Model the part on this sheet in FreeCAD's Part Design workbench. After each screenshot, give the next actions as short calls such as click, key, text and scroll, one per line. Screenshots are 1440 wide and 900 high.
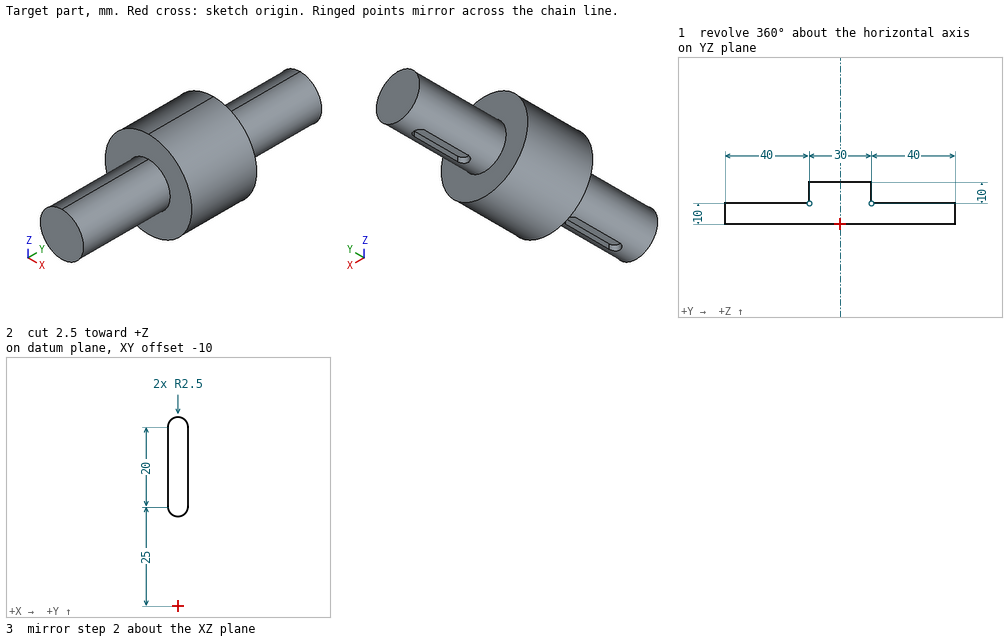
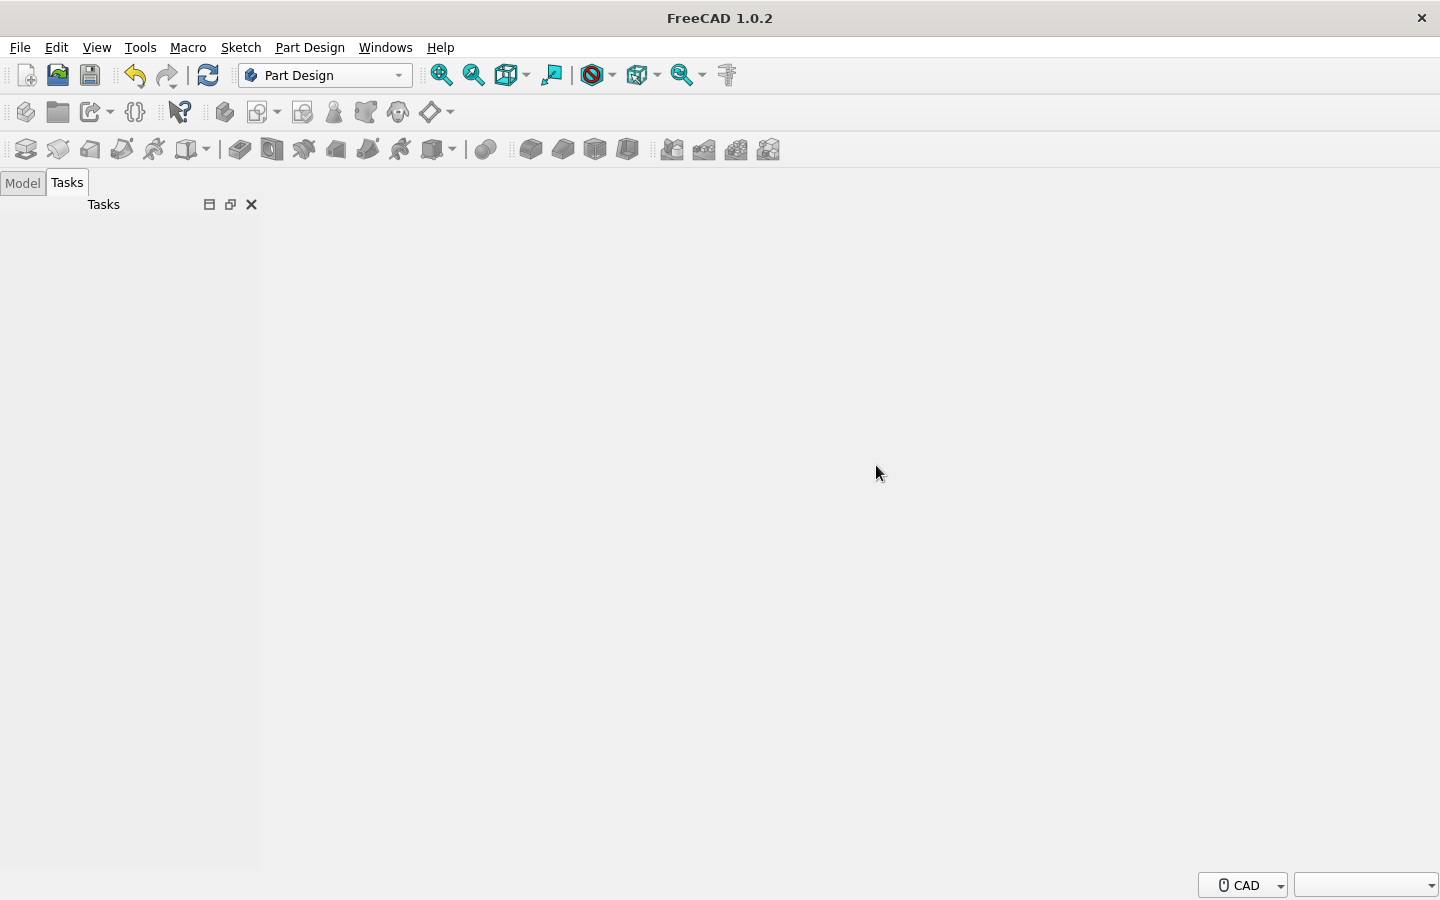
click(26, 76)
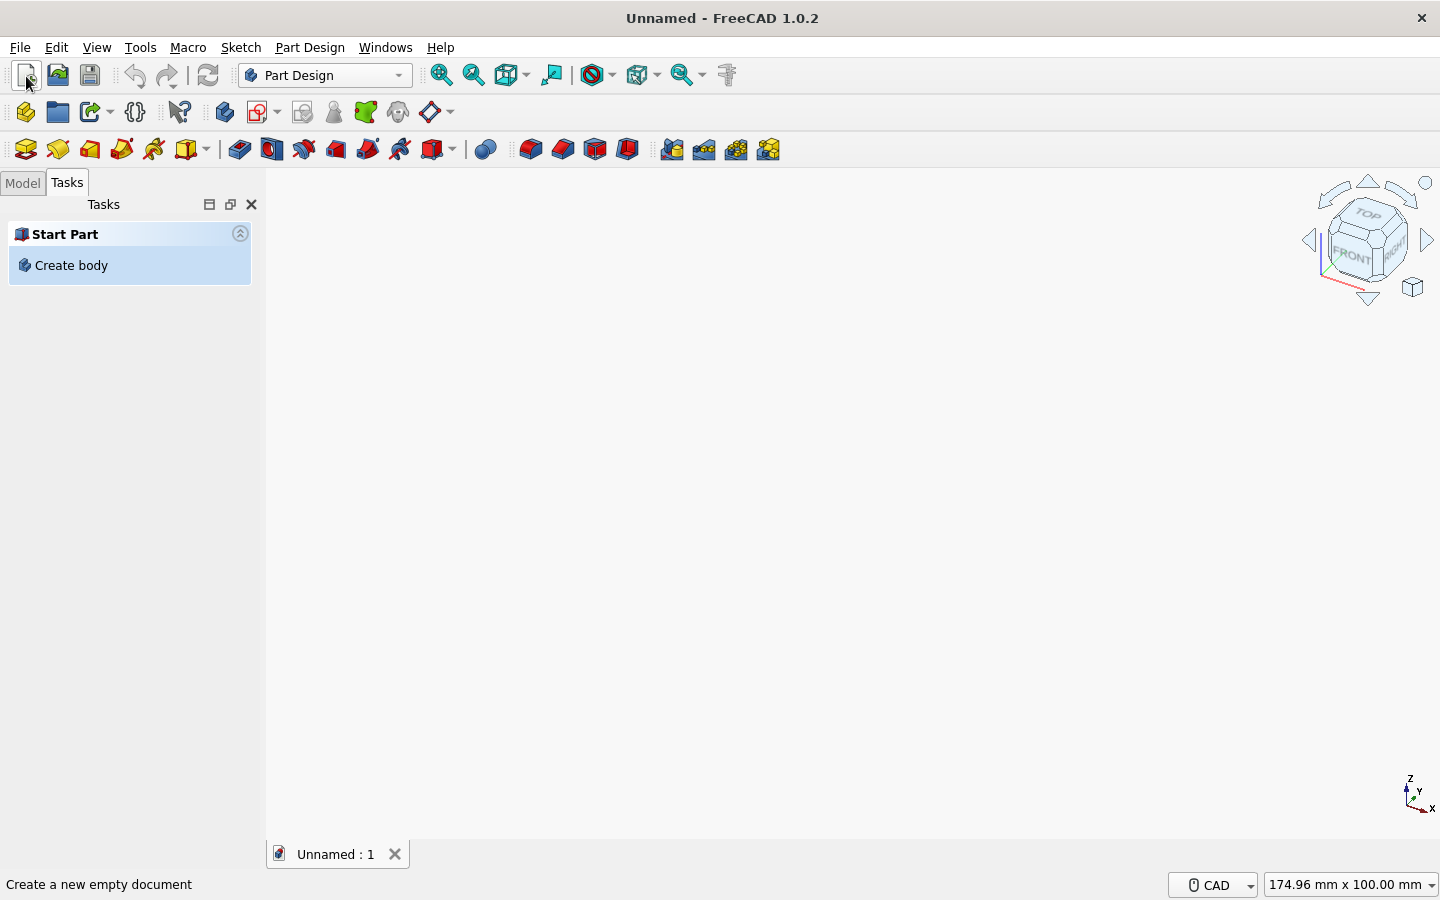
click(258, 112)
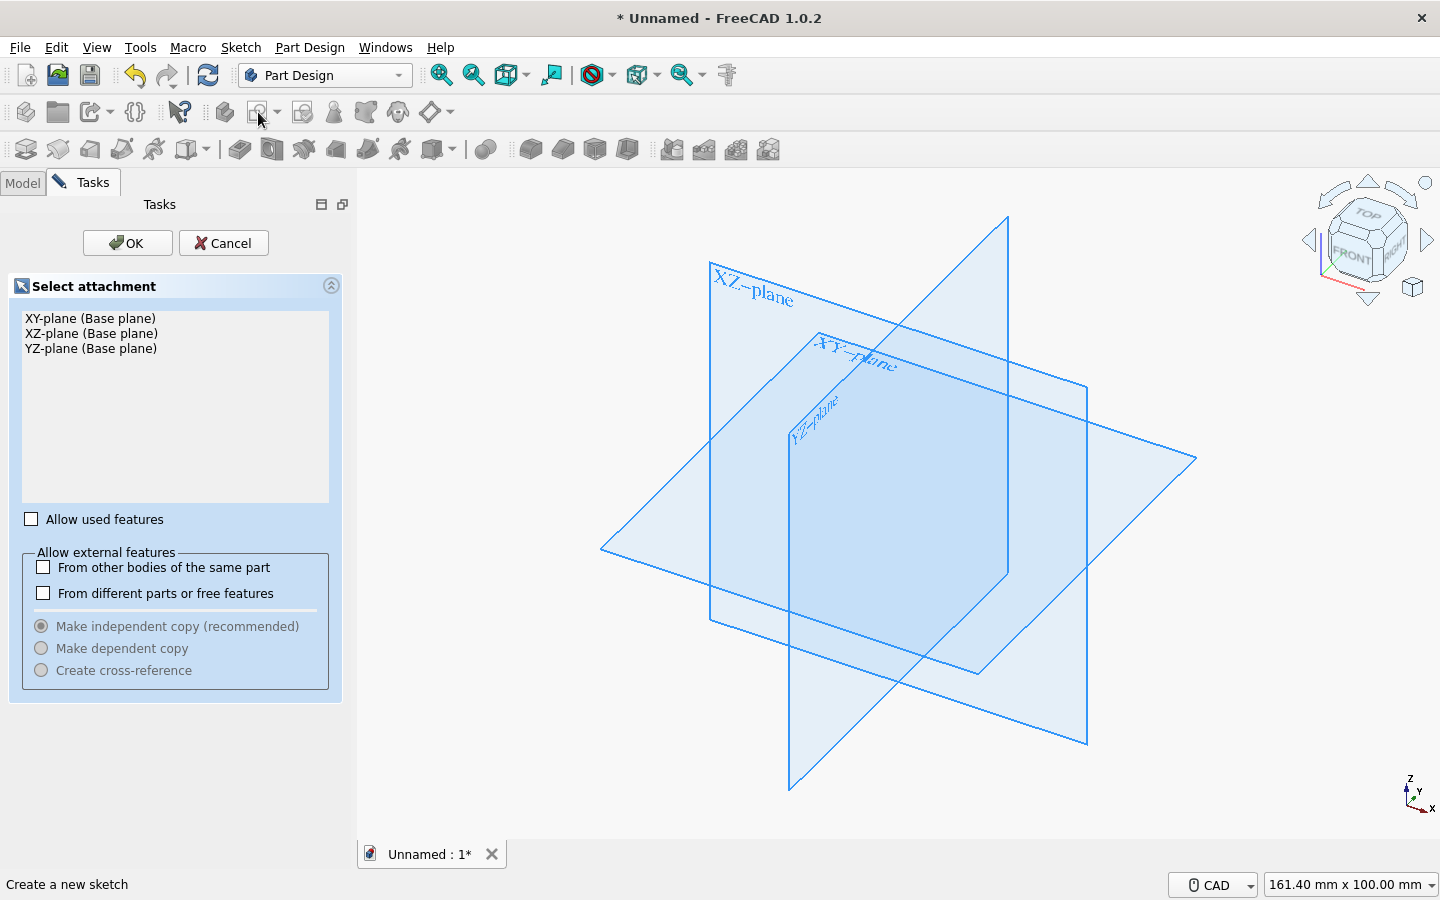
click(82, 348)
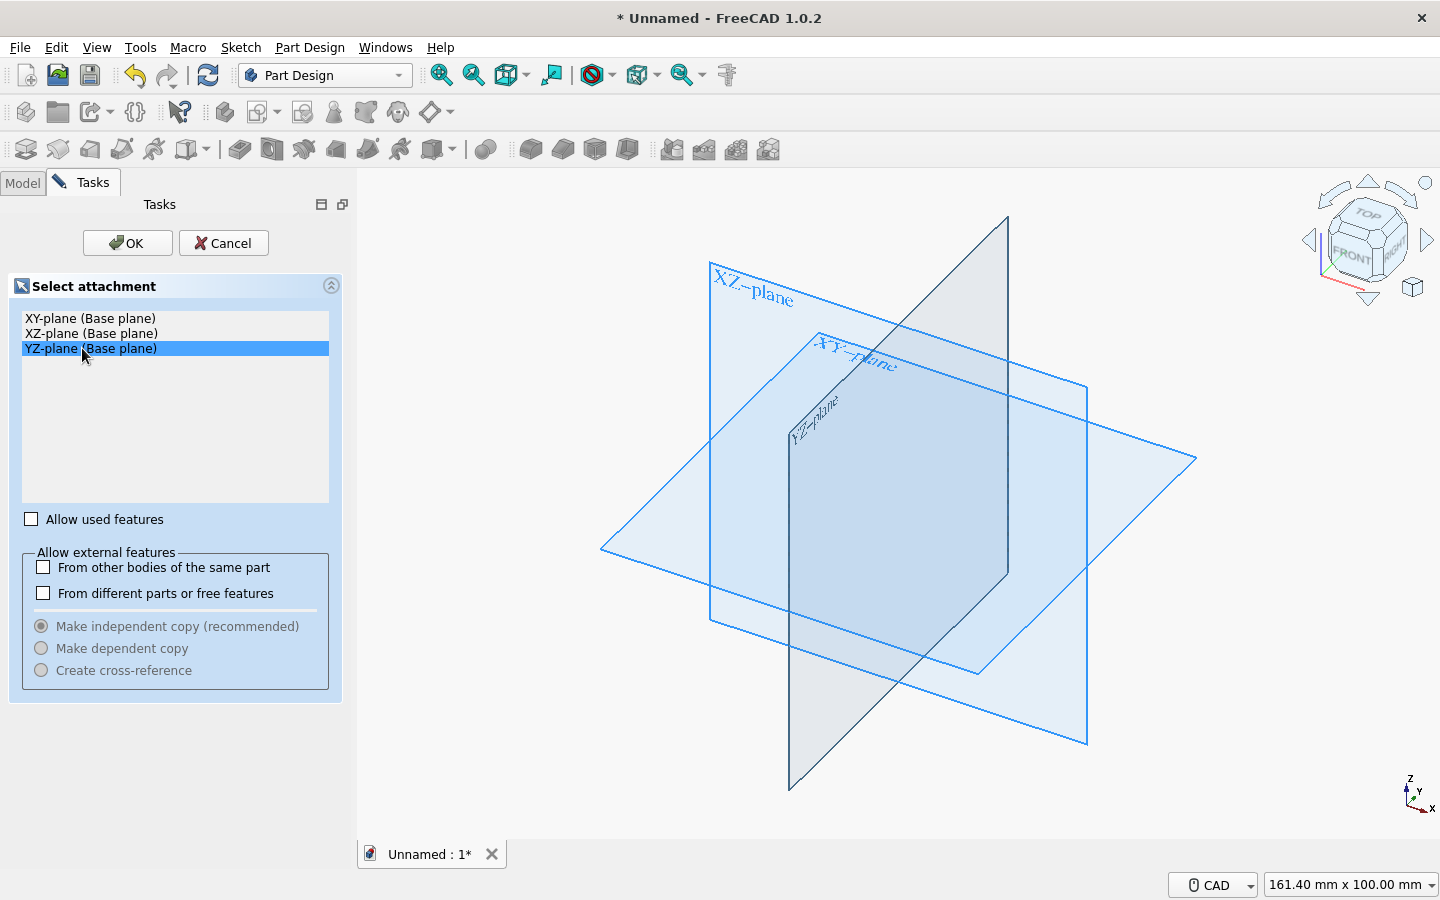
click(128, 243)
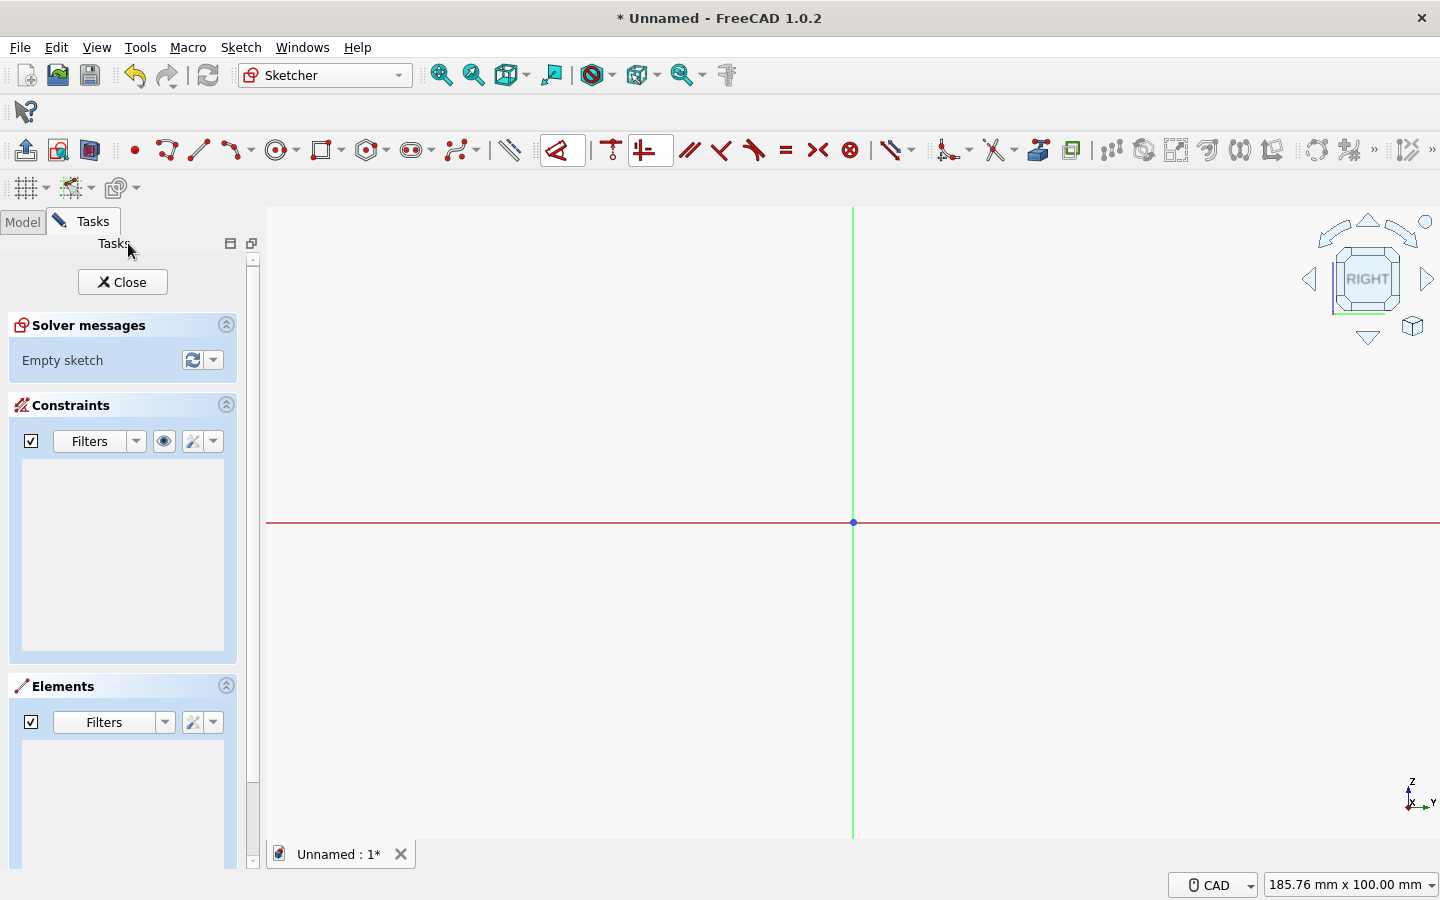
click(168, 150)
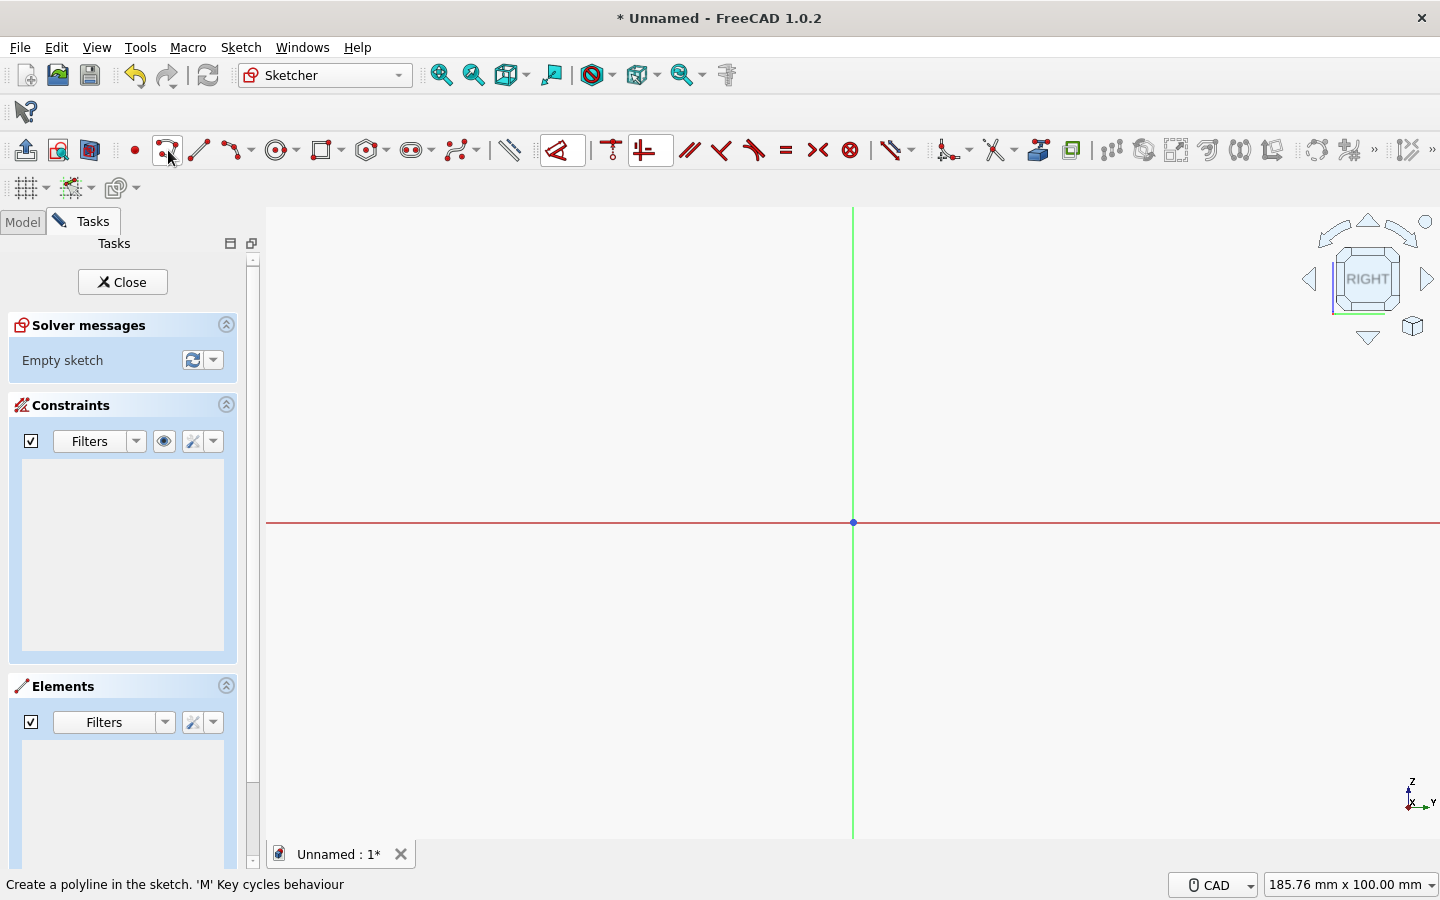
click(948, 460)
click(948, 397)
click(758, 397)
click(758, 460)
click(505, 460)
click(505, 523)
click(1201, 514)
click(1201, 460)
click(948, 461)
key(Escape)
key(Escape)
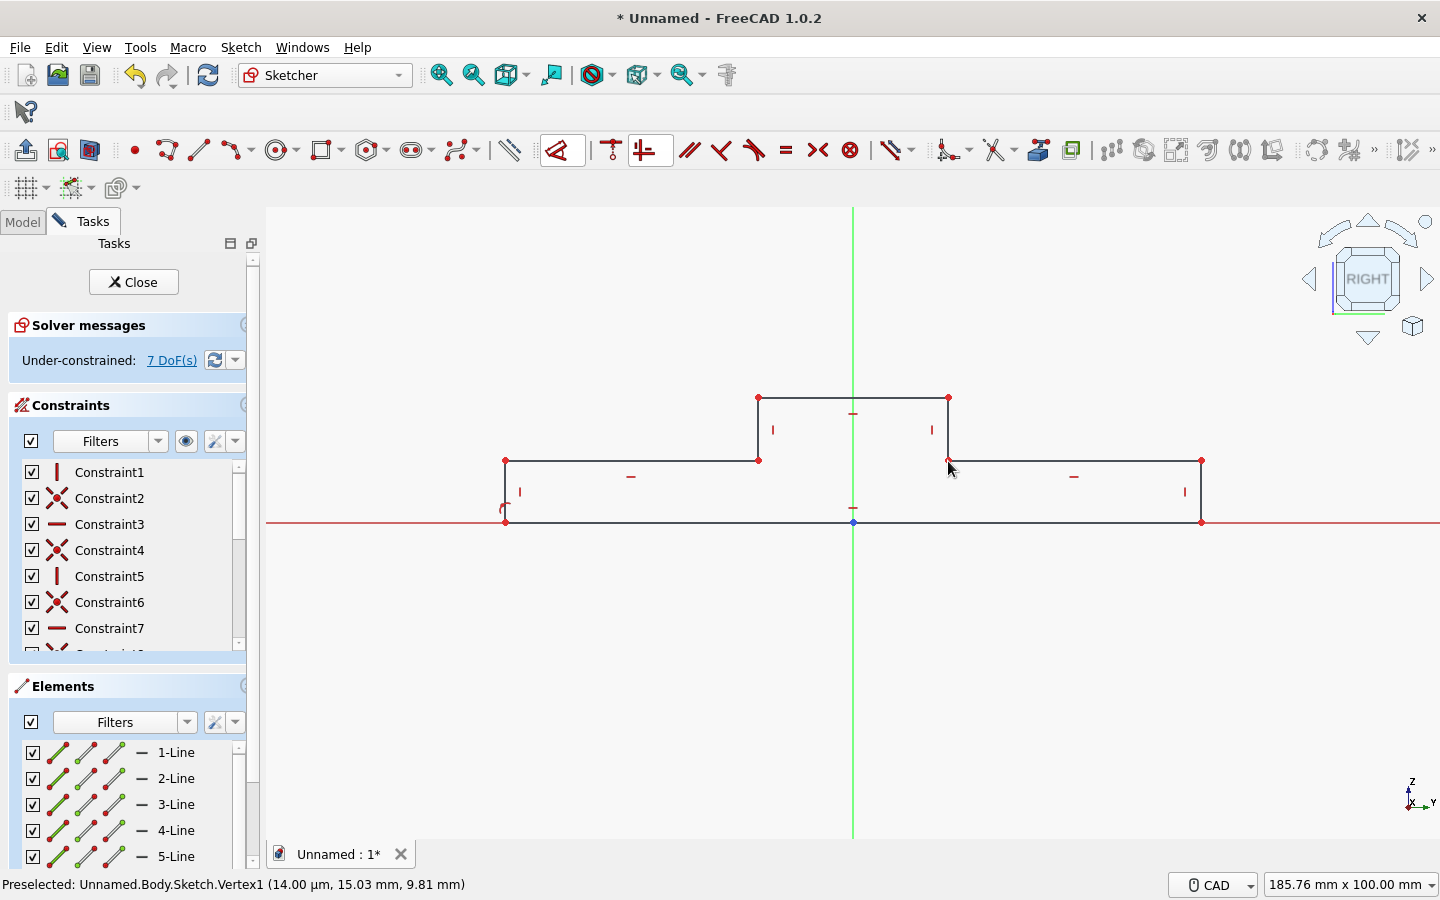
click(948, 461)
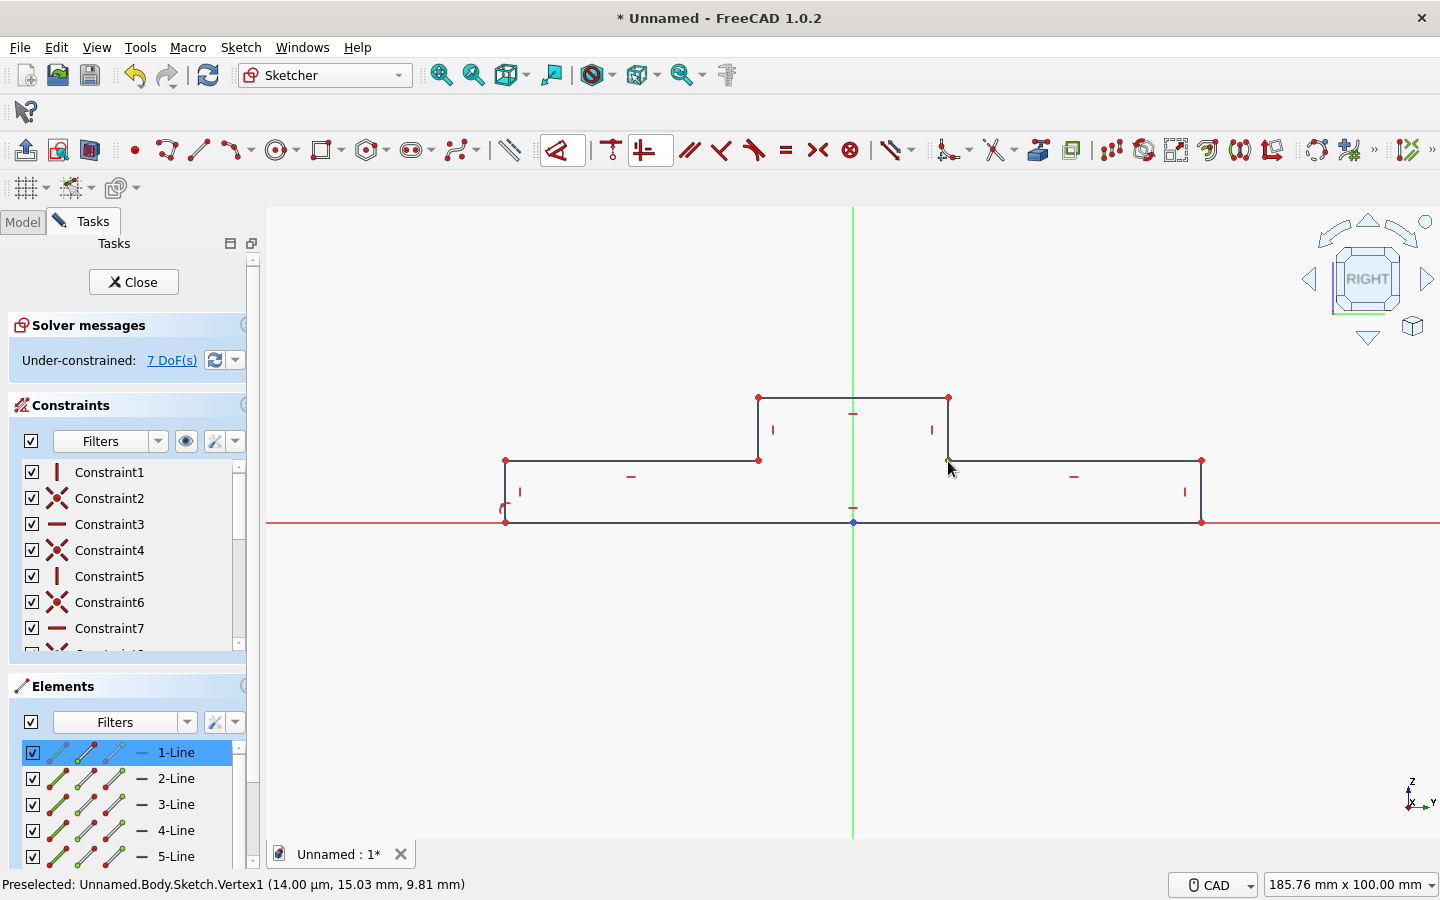
click(758, 461)